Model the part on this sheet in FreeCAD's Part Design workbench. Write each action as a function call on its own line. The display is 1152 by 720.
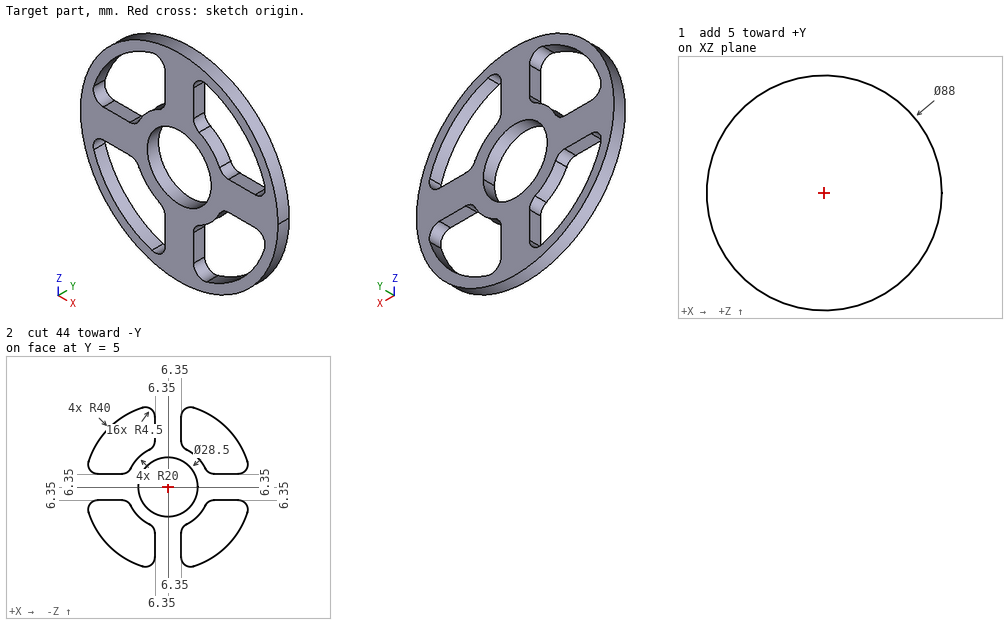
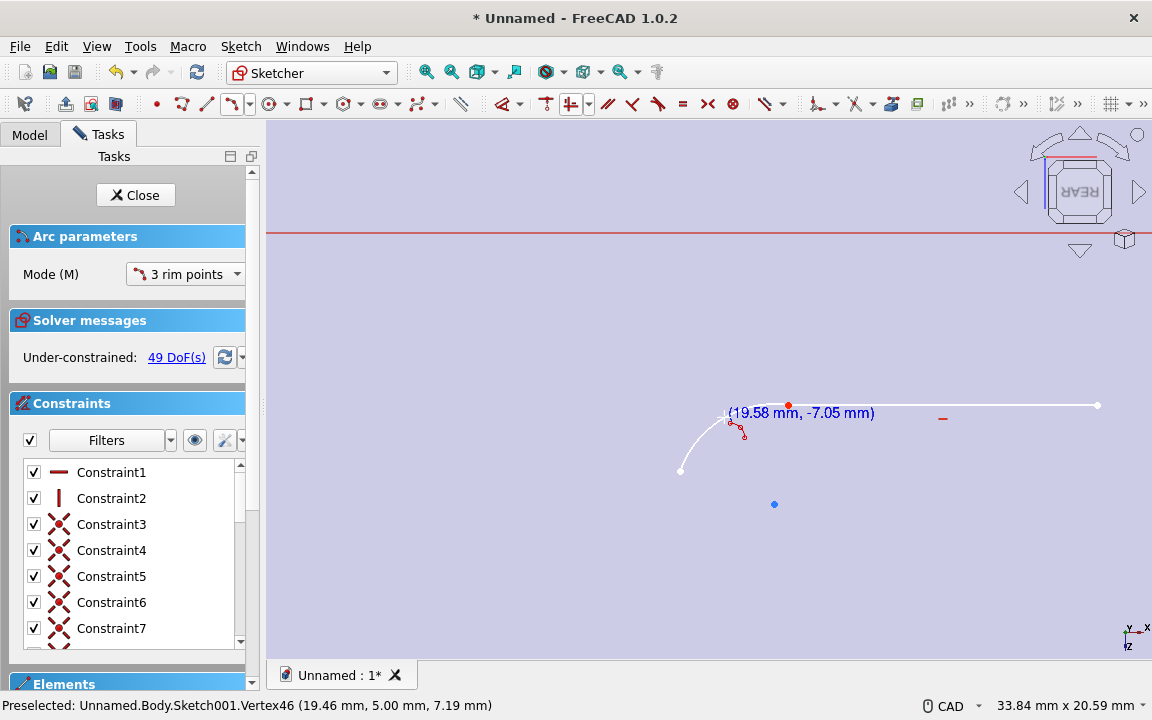
scroll(725, 420, down, 9)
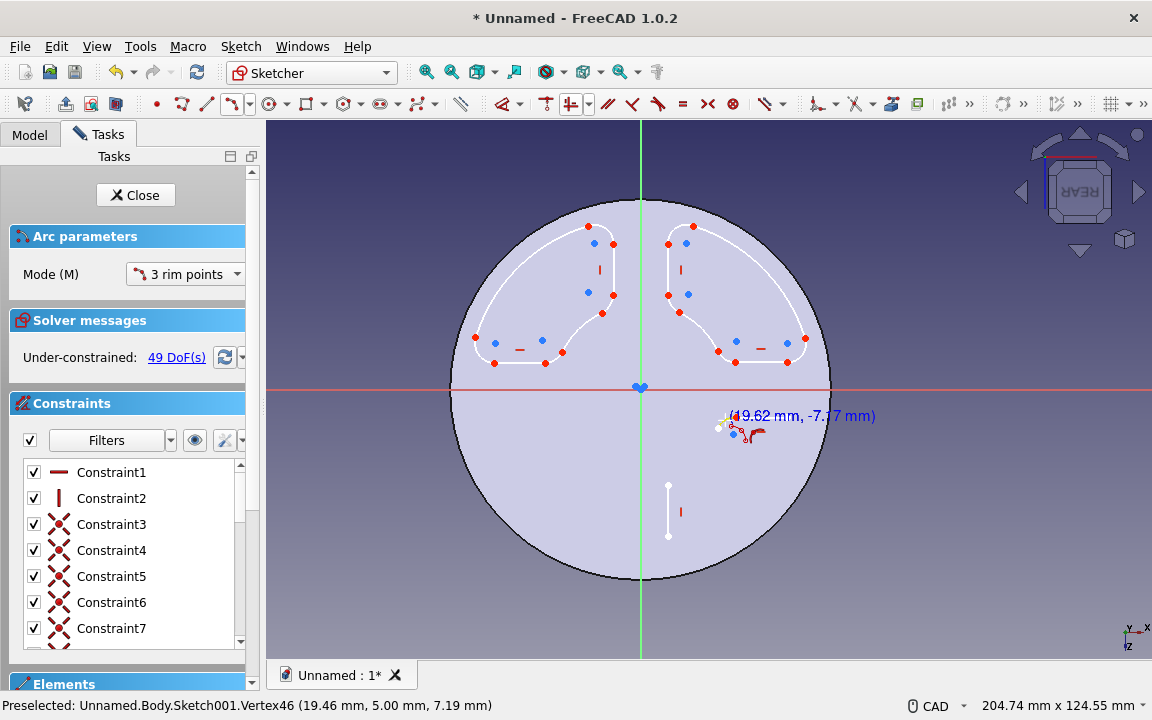
click(718, 429)
click(679, 467)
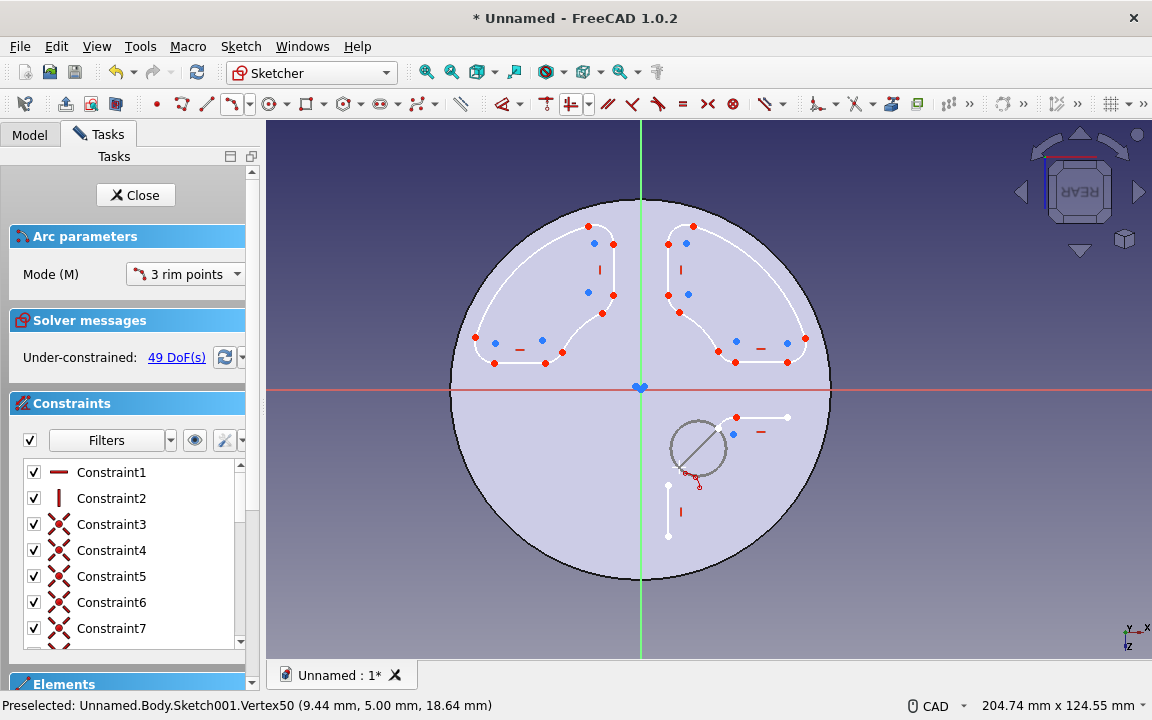
scroll(702, 451, up, 7)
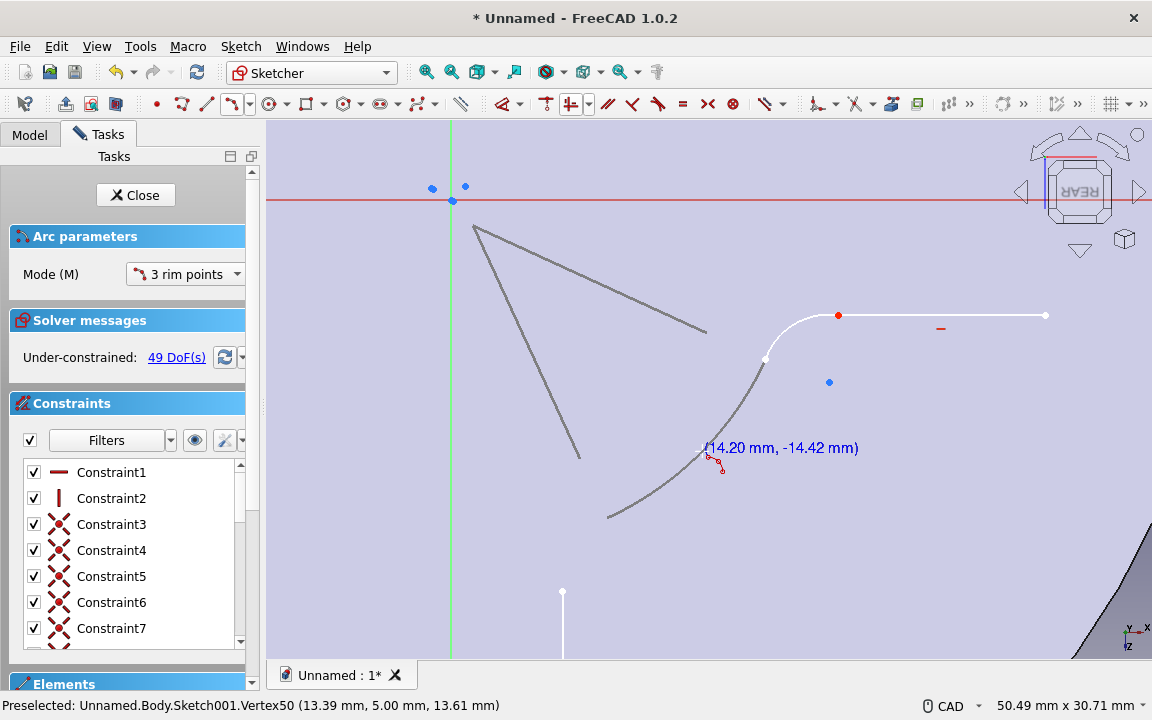
click(699, 448)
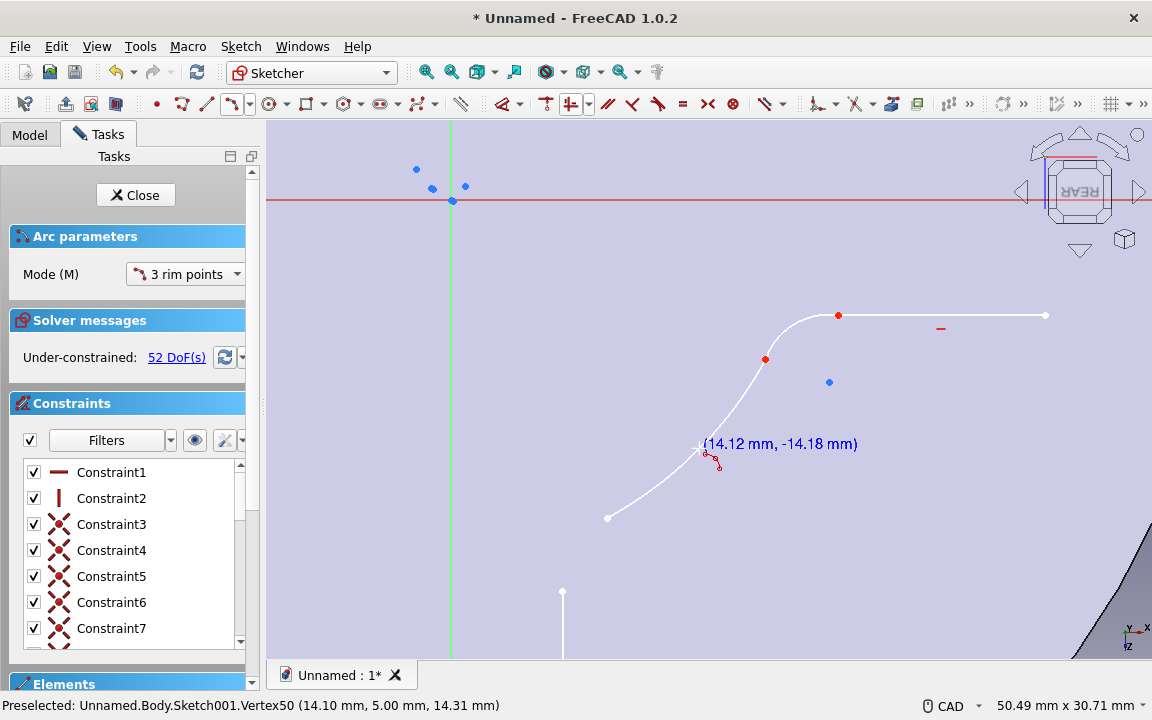
scroll(702, 451, down, 7)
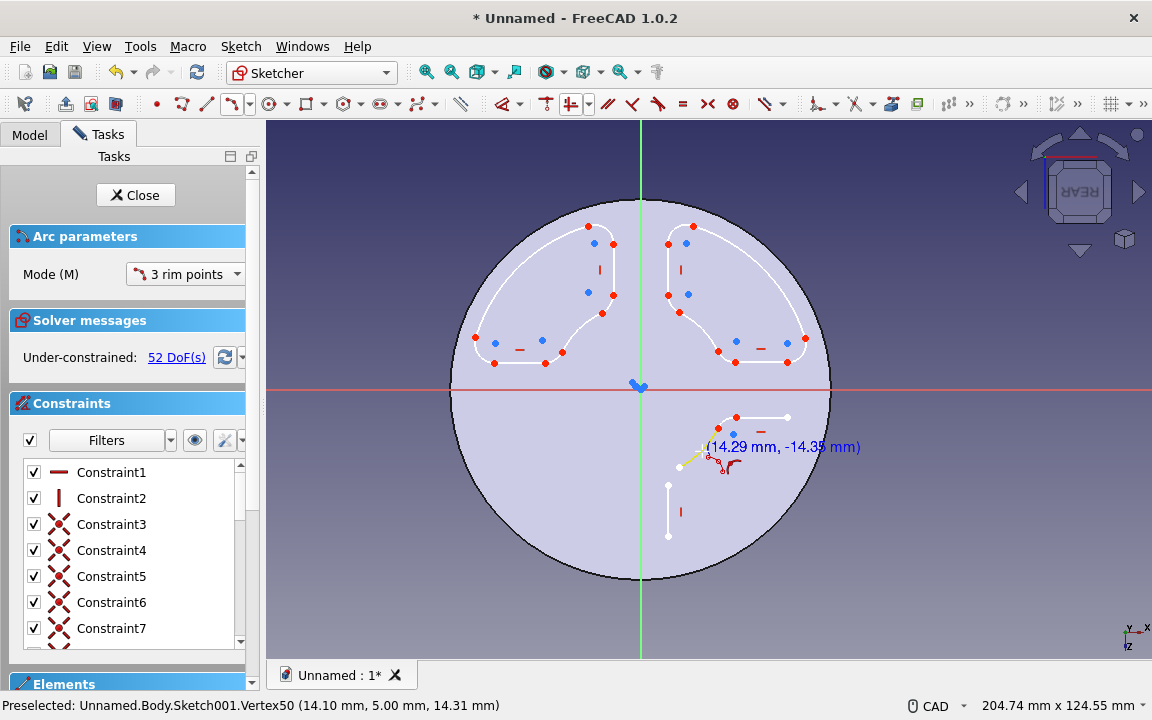
click(679, 468)
click(668, 486)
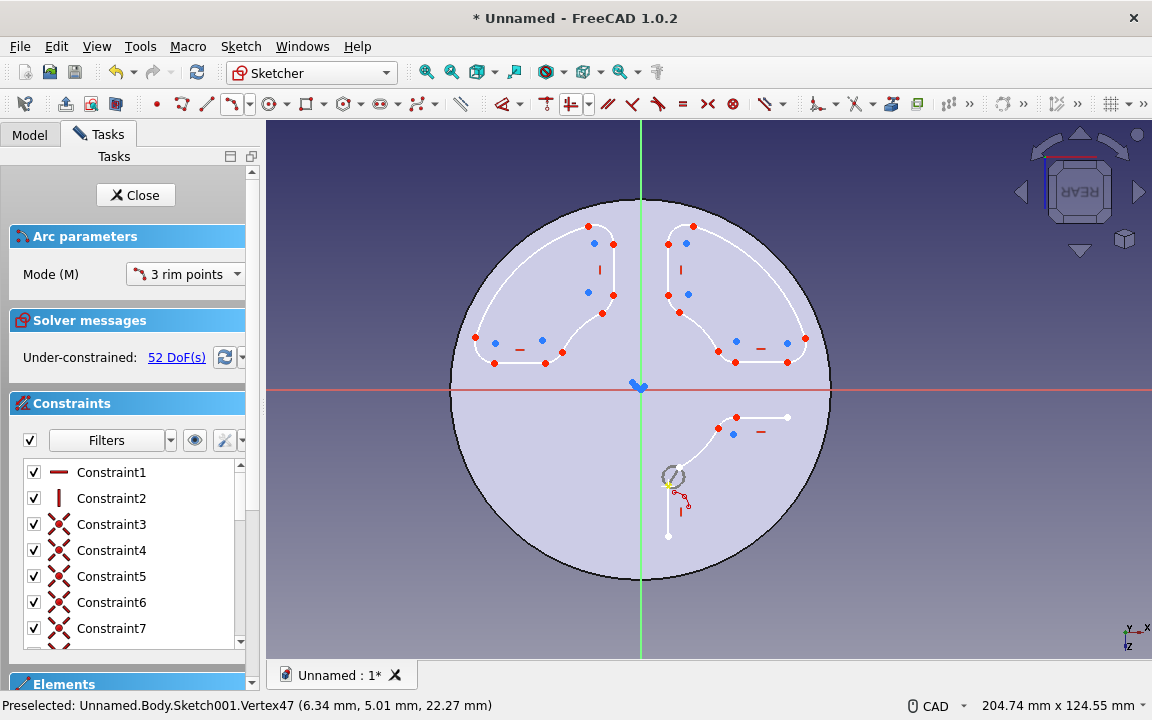
scroll(671, 474, up, 9)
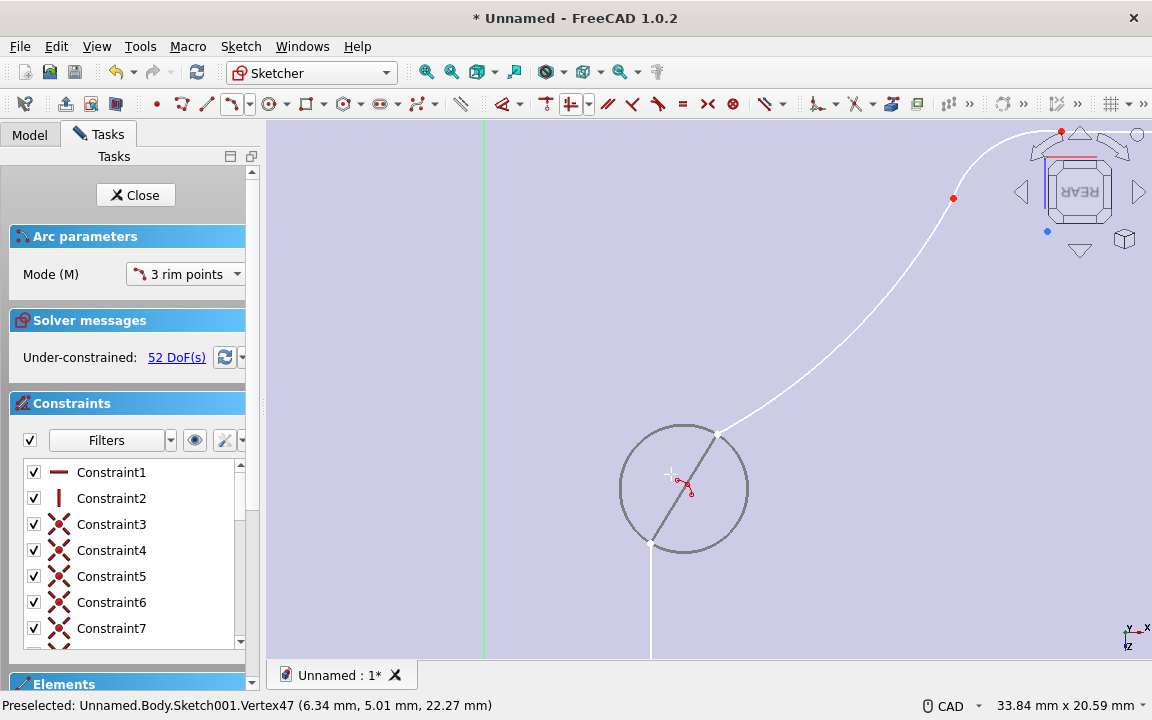
click(668, 473)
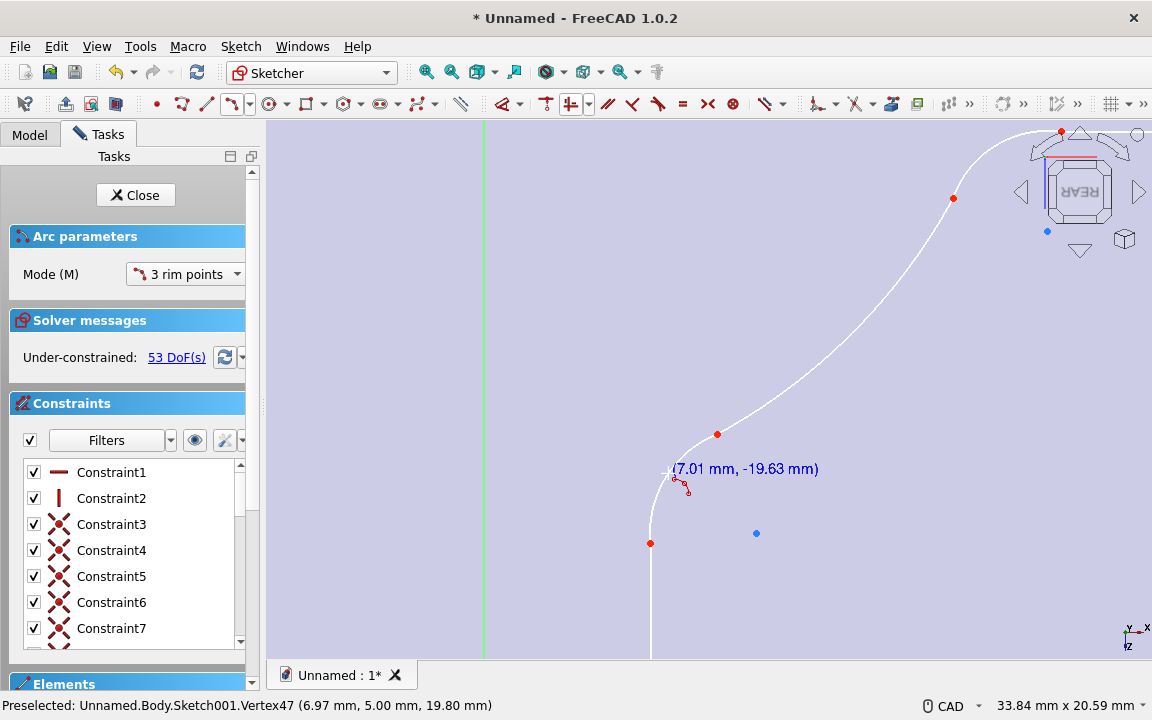
scroll(671, 475, down, 9)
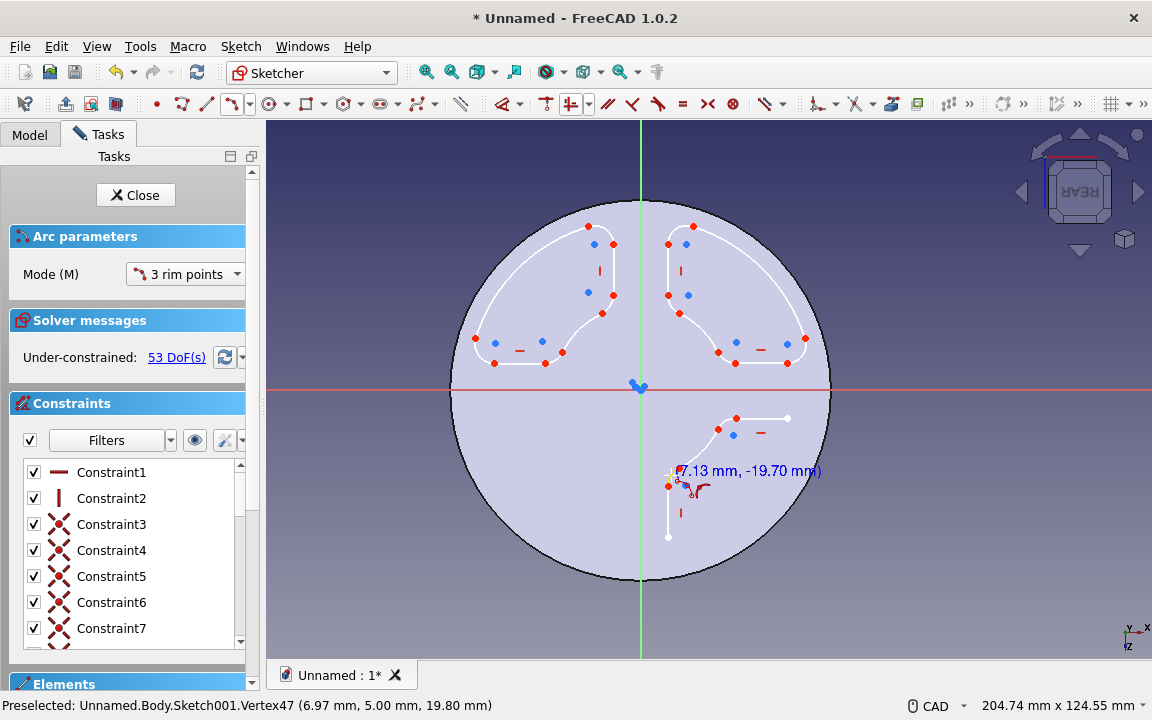
click(668, 538)
click(693, 555)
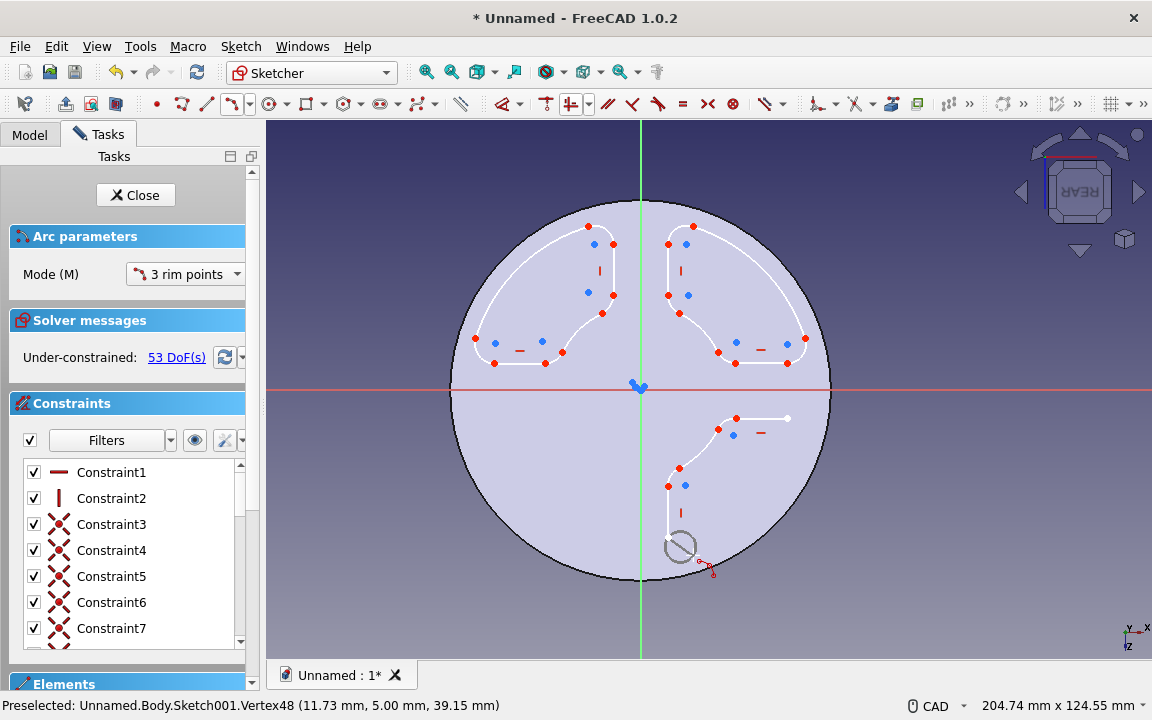
scroll(676, 552, up, 4)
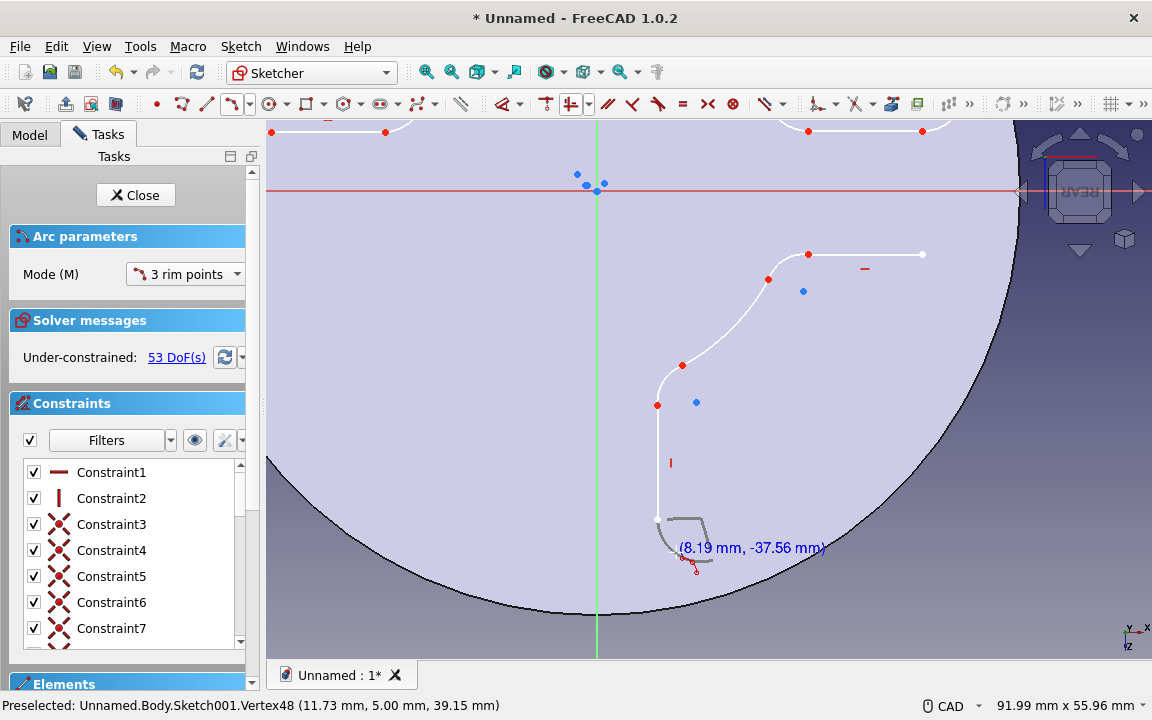
click(675, 552)